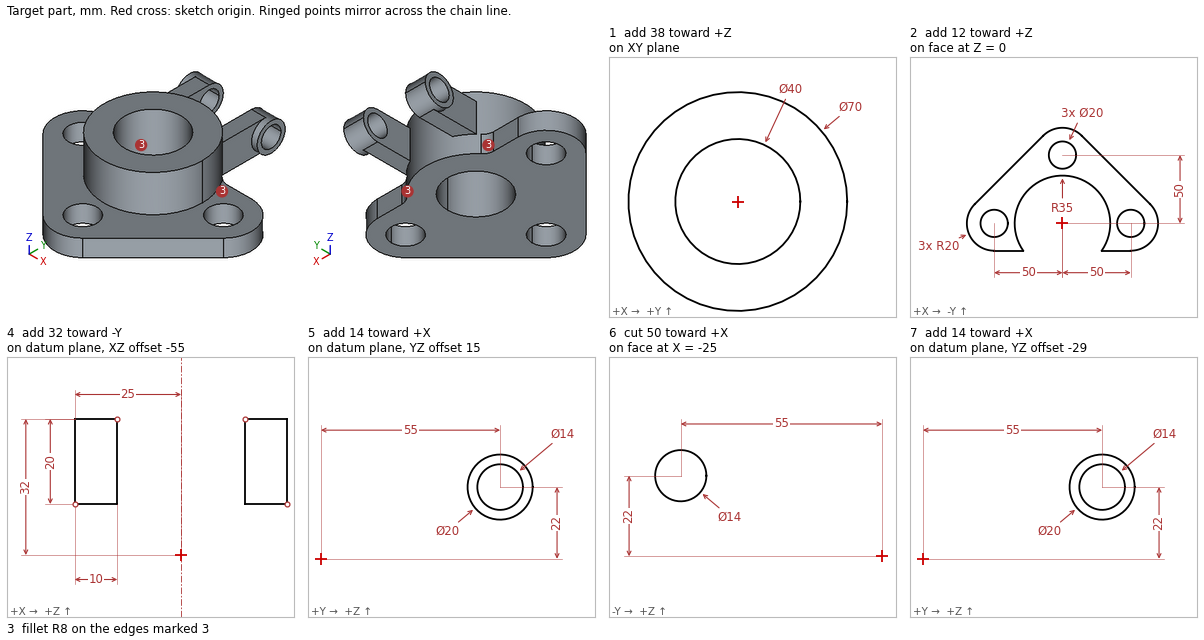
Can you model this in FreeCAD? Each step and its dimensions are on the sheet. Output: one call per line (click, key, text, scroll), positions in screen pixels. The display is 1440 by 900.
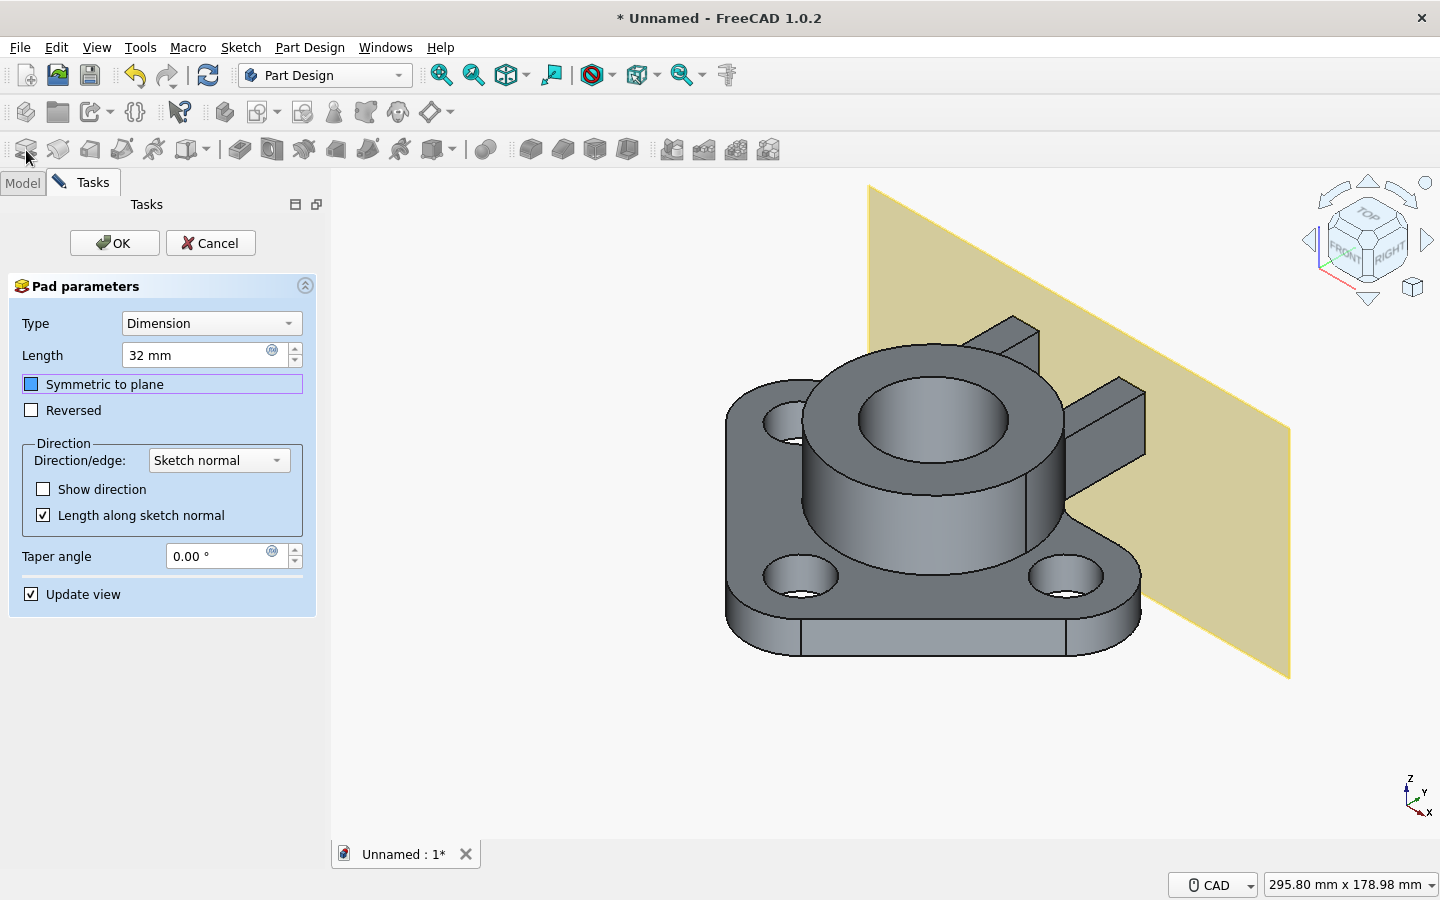
click(115, 243)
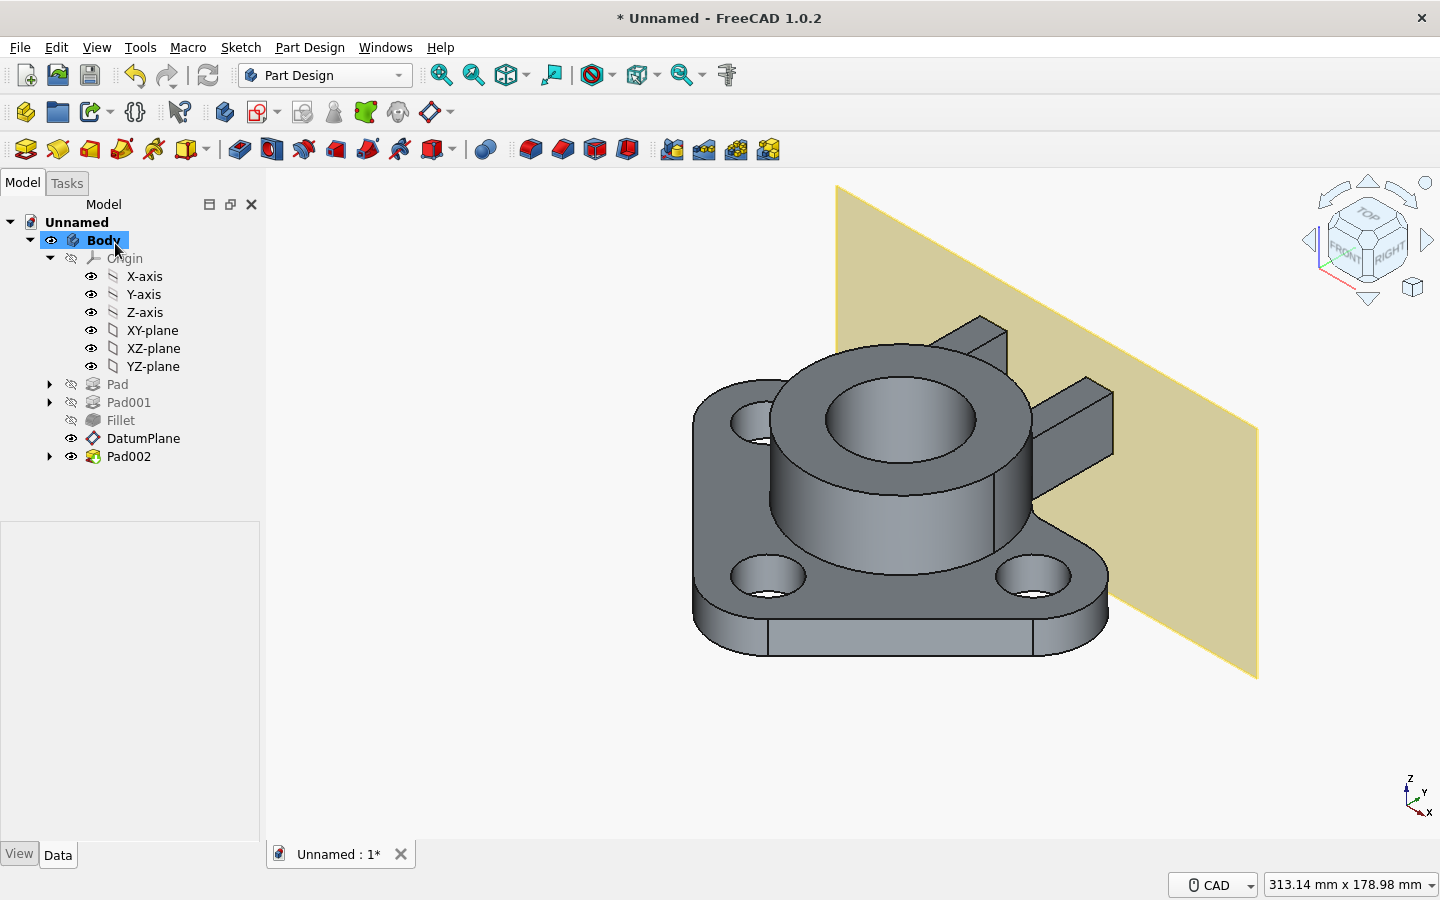
click(116, 438)
key(space)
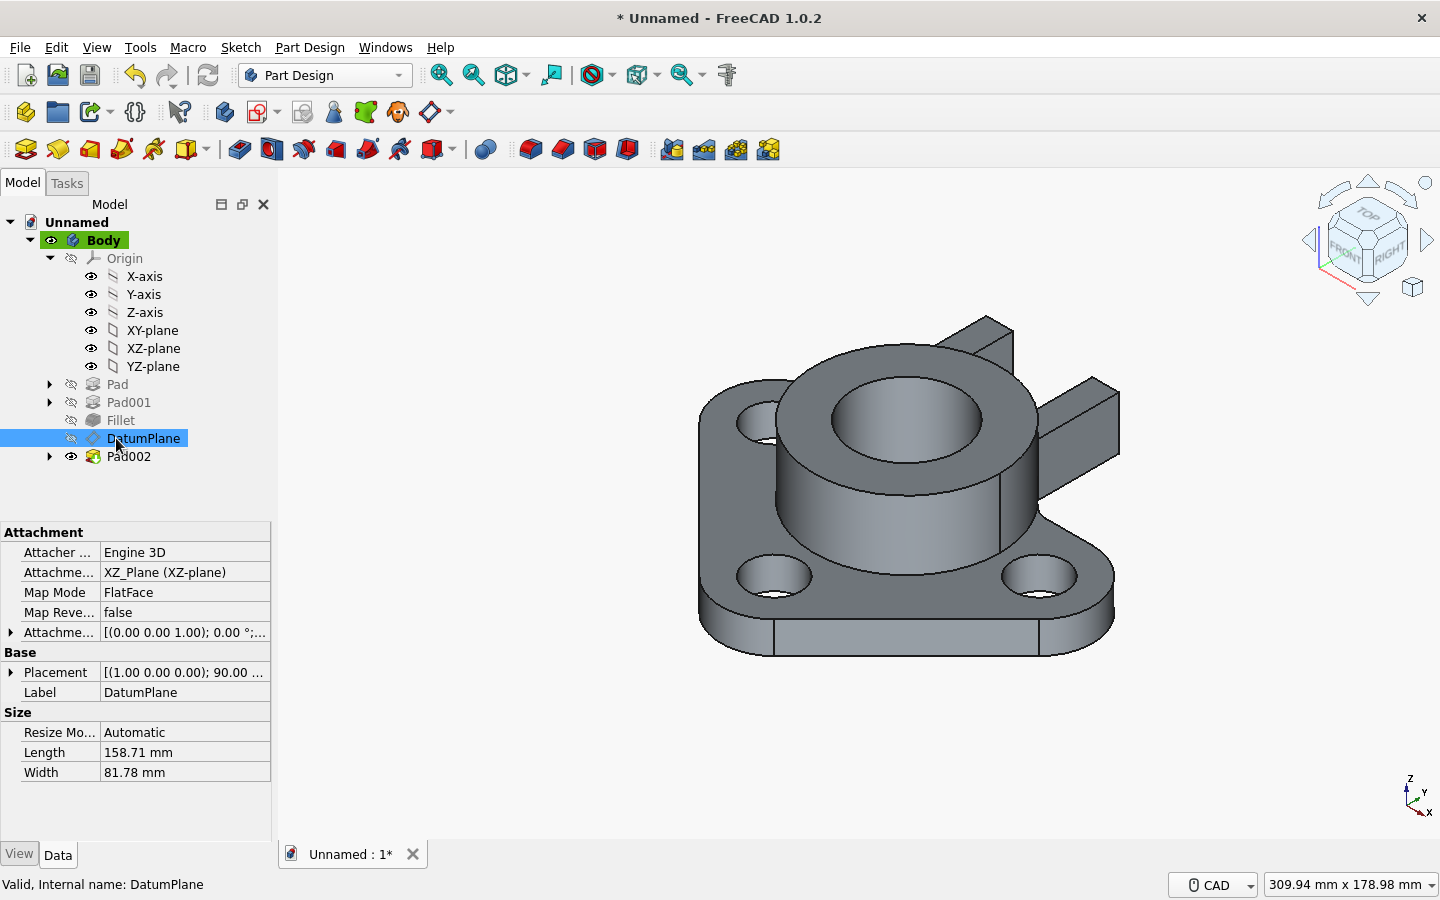
click(136, 366)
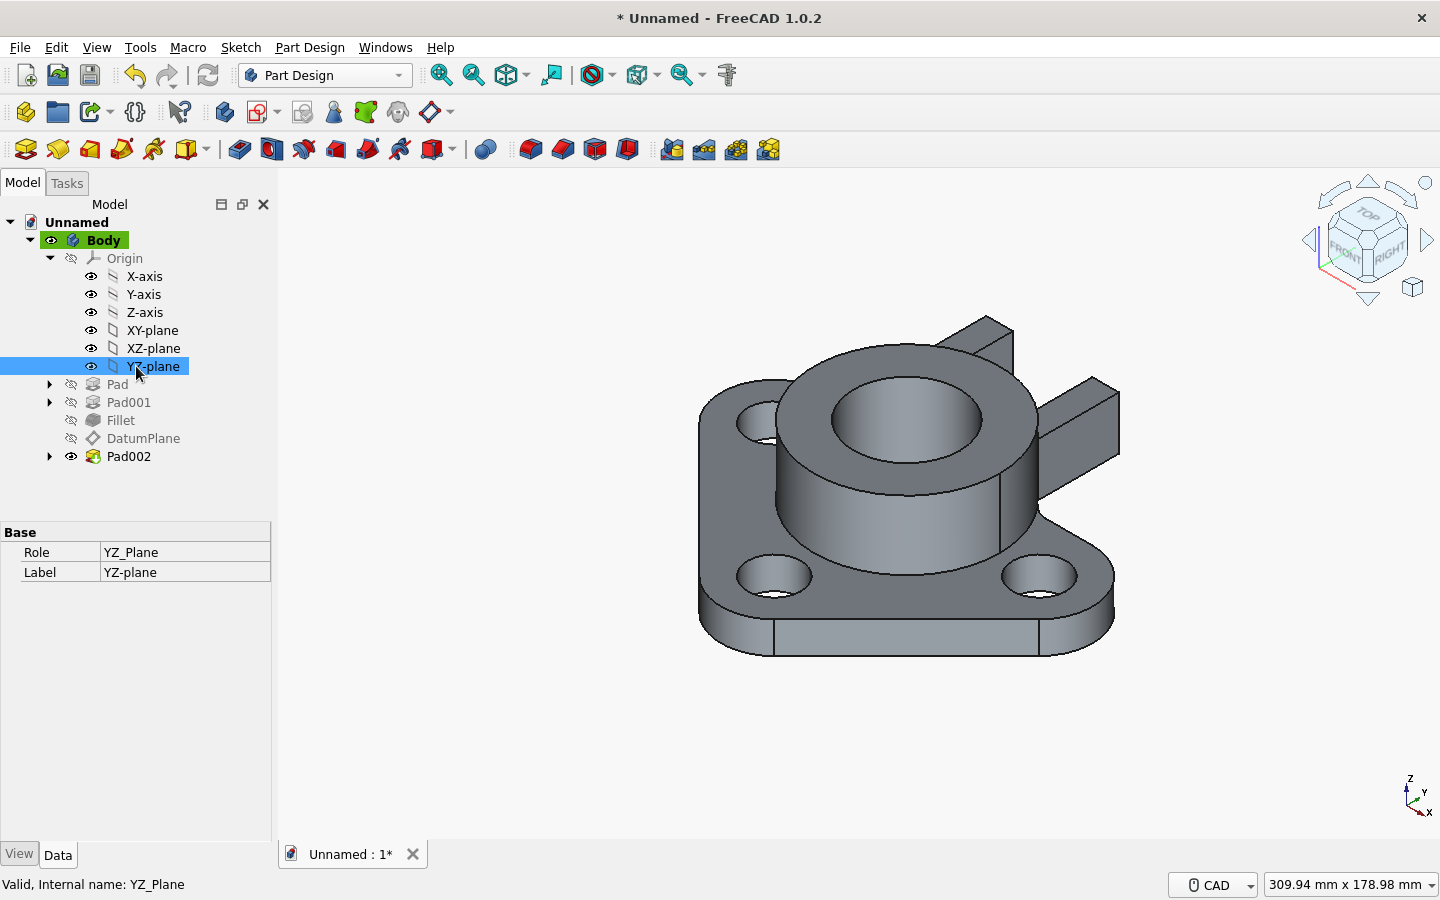
click(430, 112)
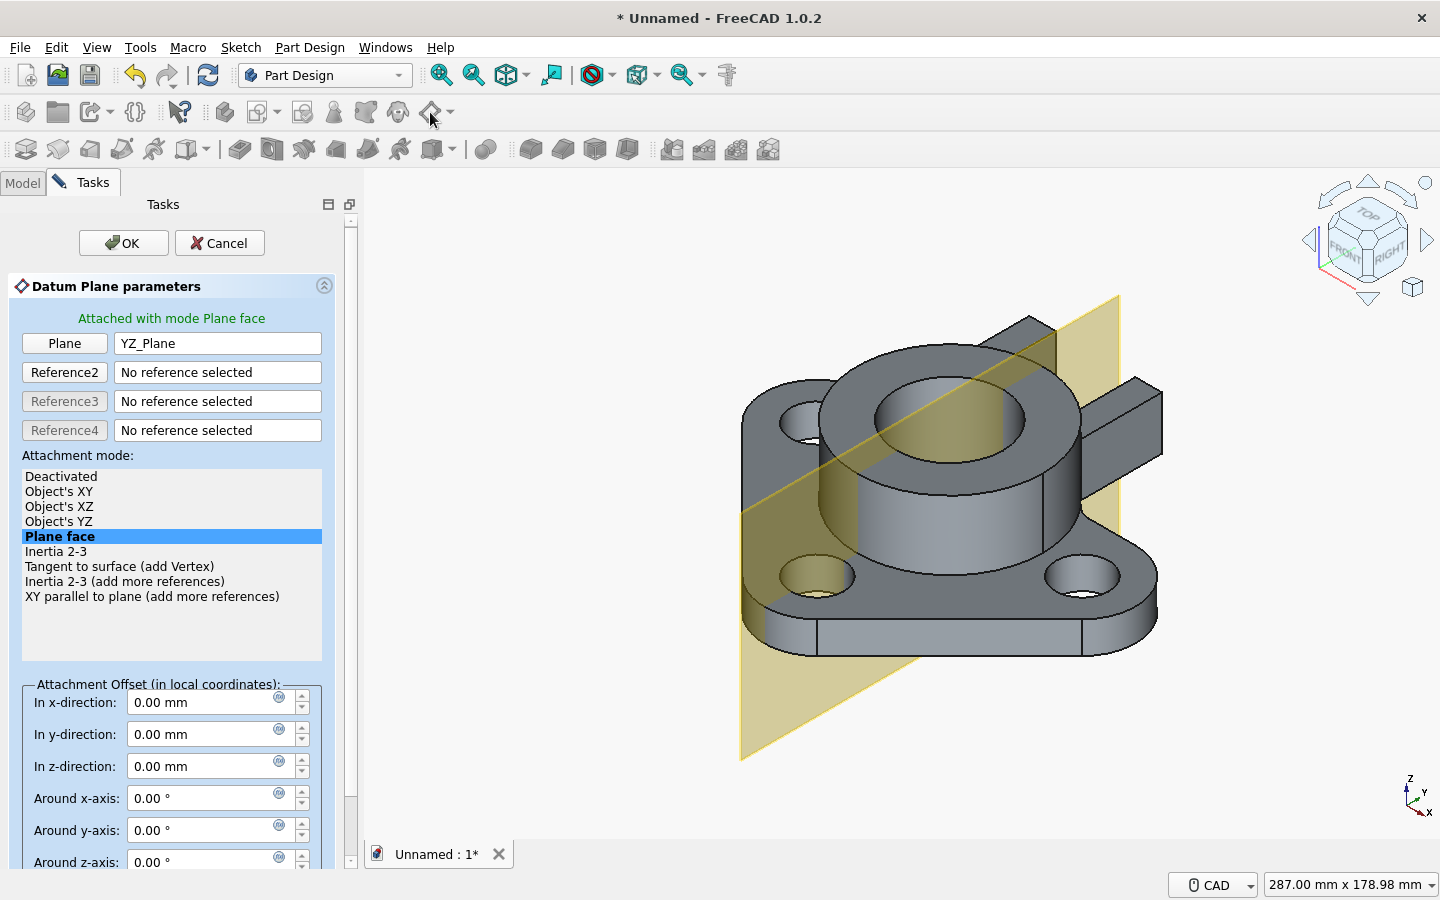
triple_click(210, 766)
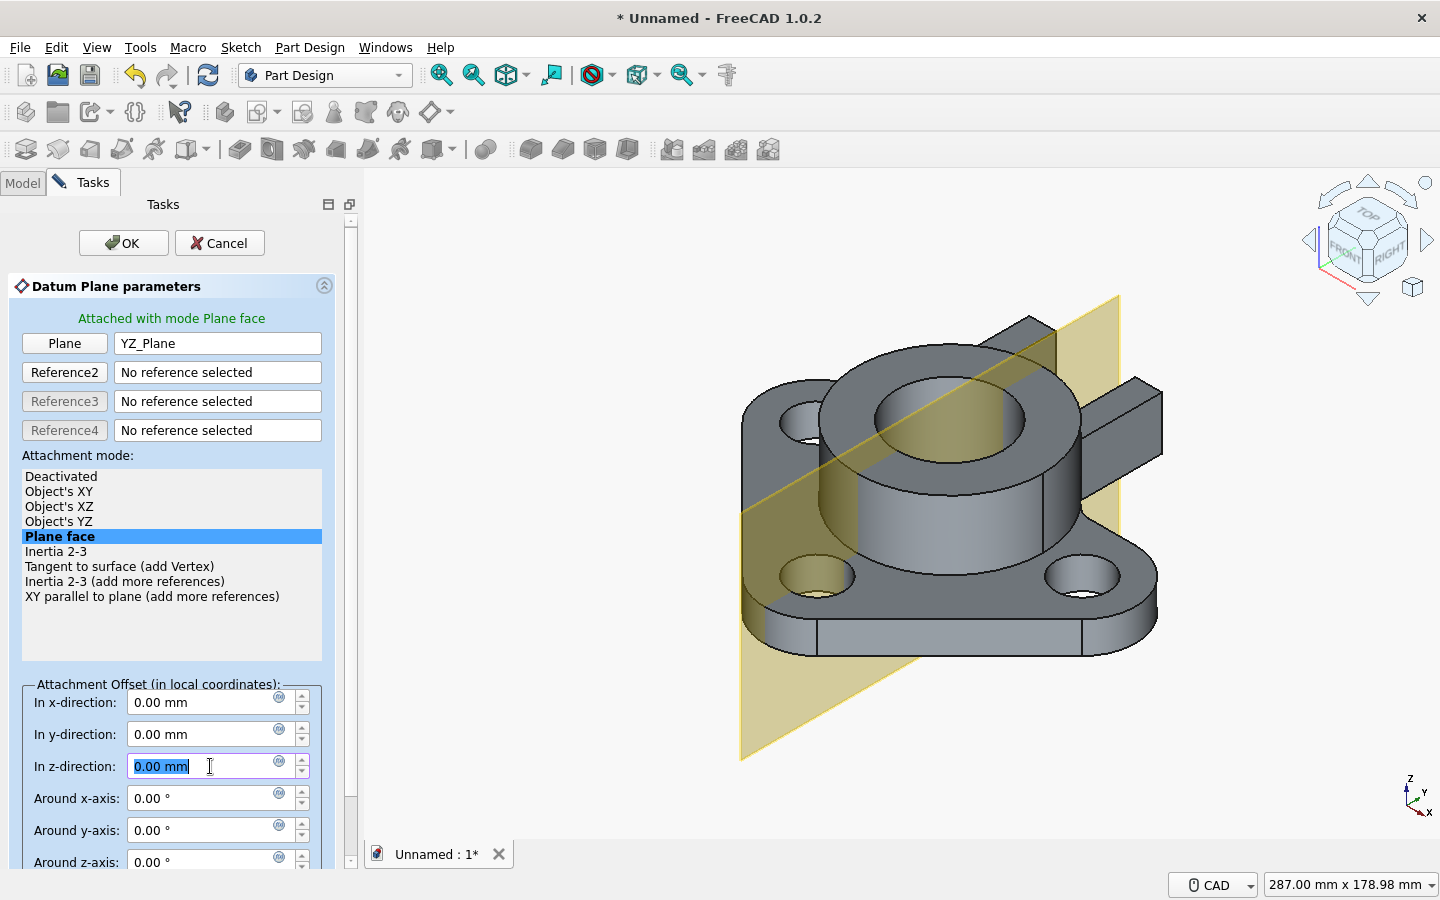
text(15)
key(Tab)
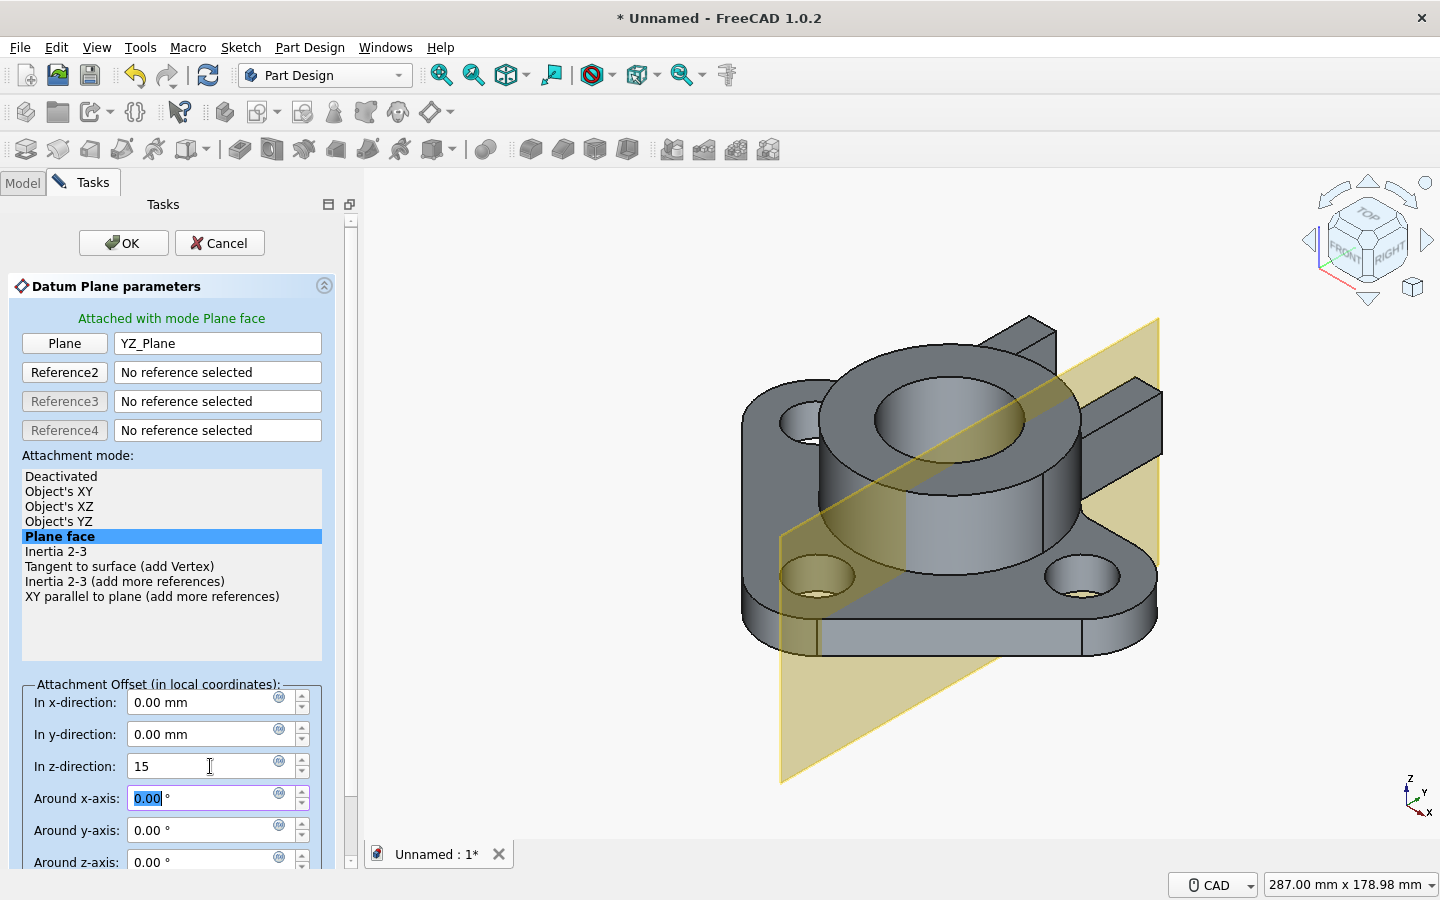
click(124, 243)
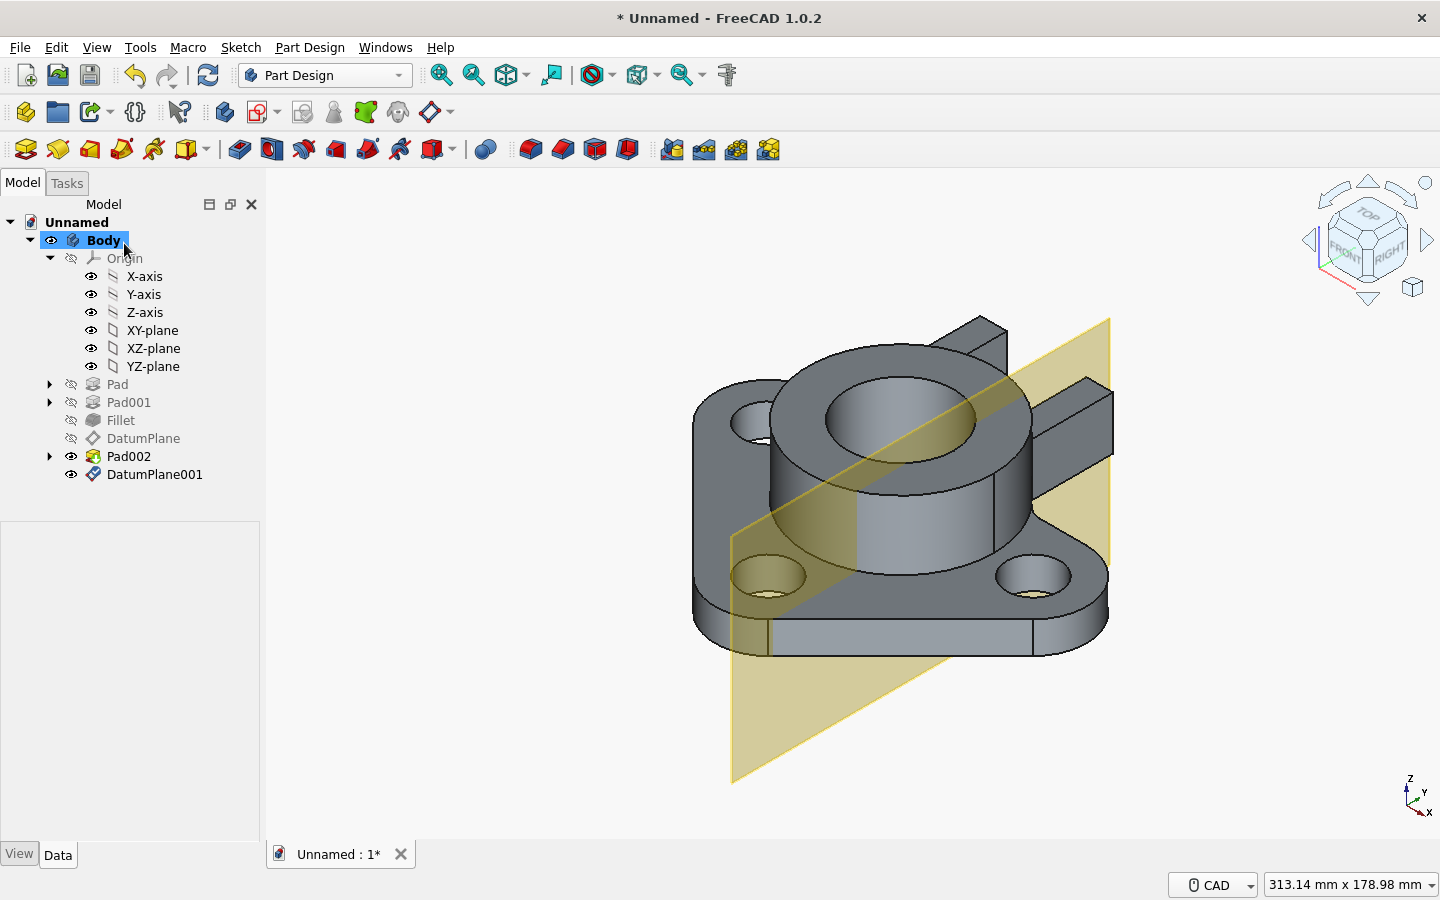
click(116, 474)